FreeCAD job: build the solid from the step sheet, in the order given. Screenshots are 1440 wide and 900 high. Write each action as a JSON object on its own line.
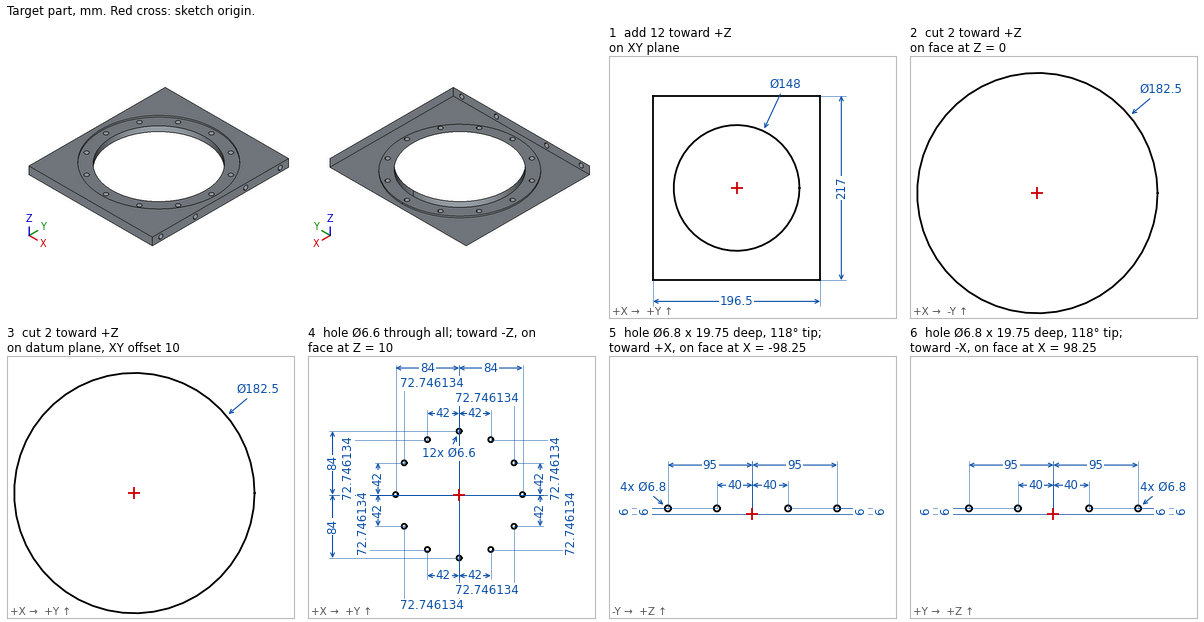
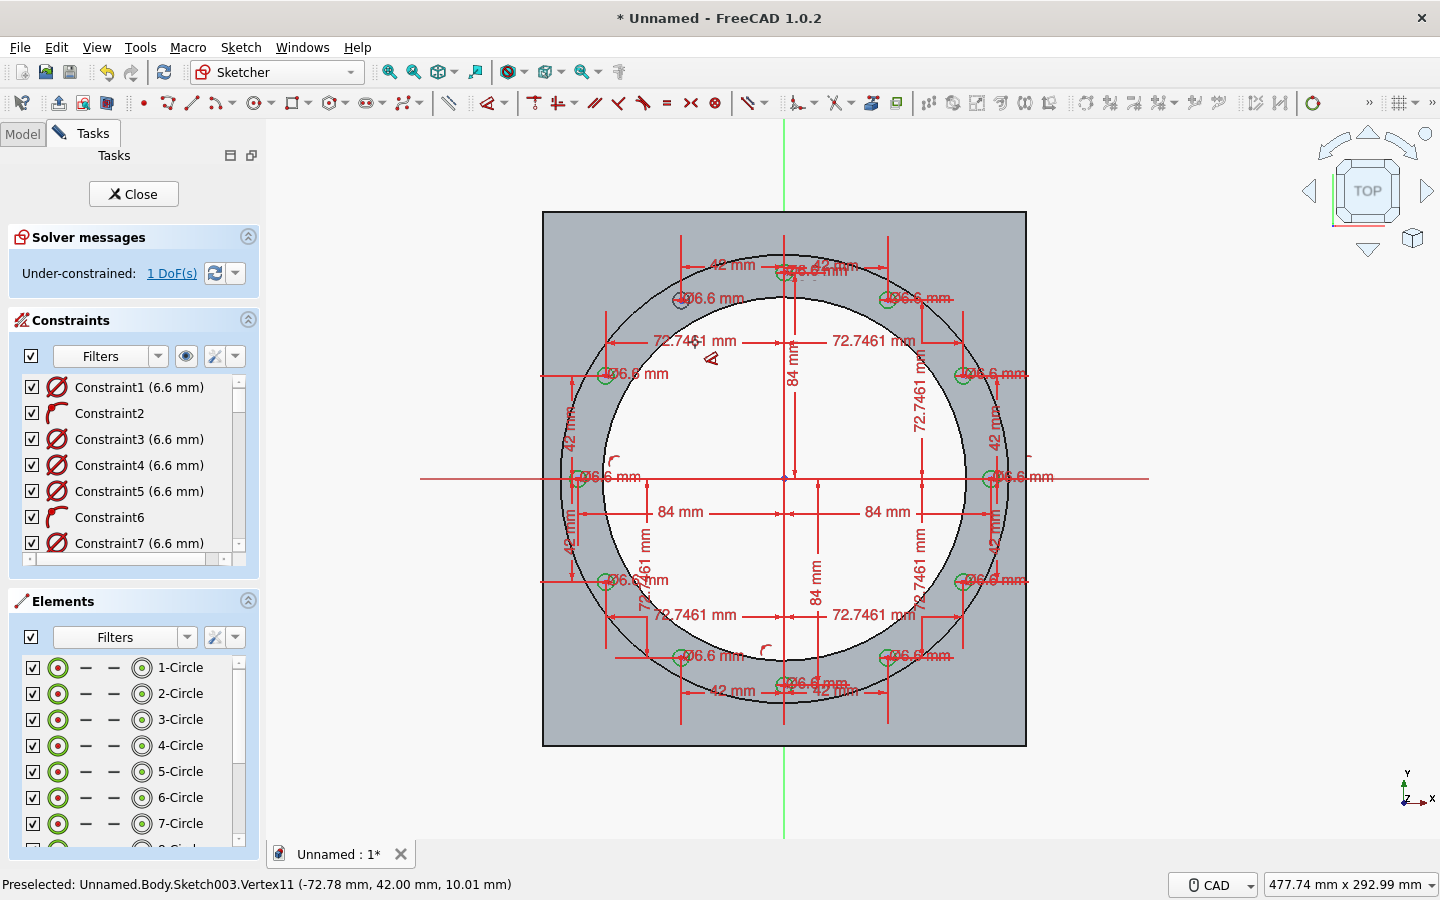
{"action": "left_click", "coordinate": [681, 300]}
{"action": "left_click", "coordinate": [647, 390]}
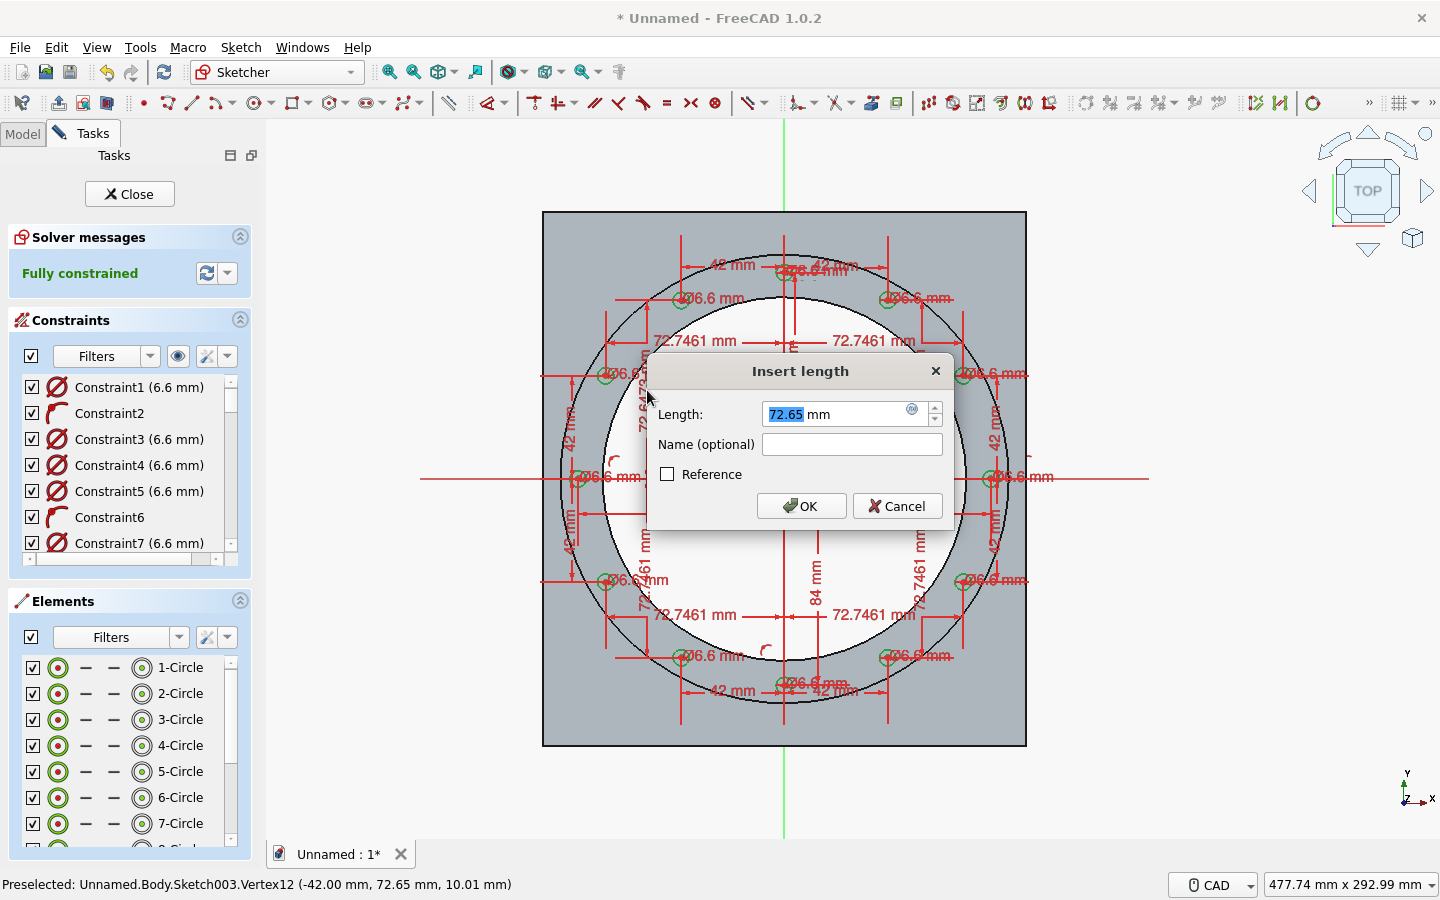
{"action": "type", "text": "72.746134"}
{"action": "key", "text": "Return"}
{"action": "key", "text": "Escape"}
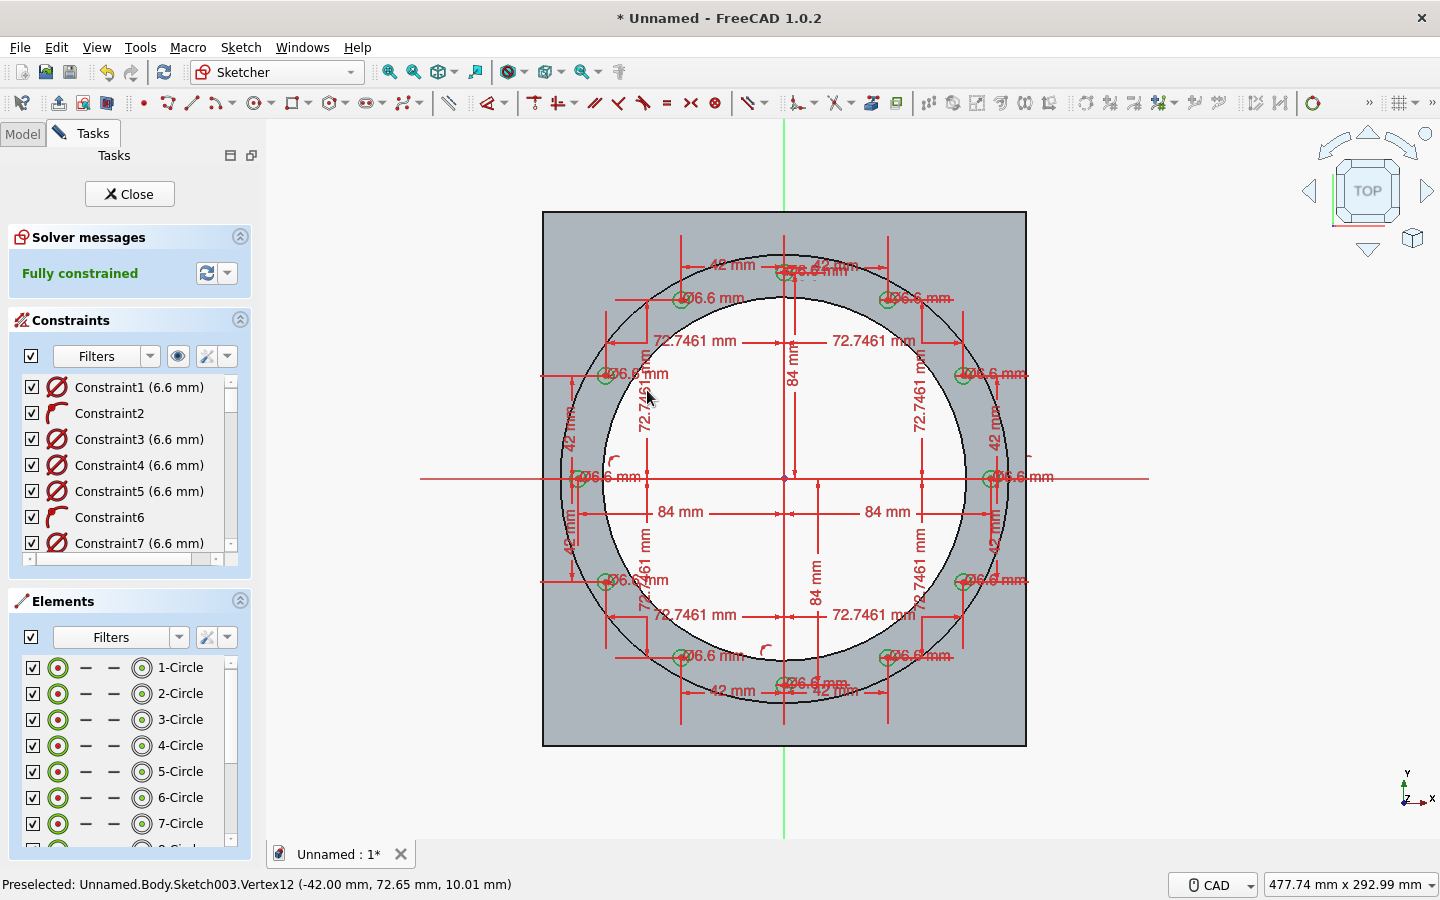
{"action": "left_click", "coordinate": [130, 194]}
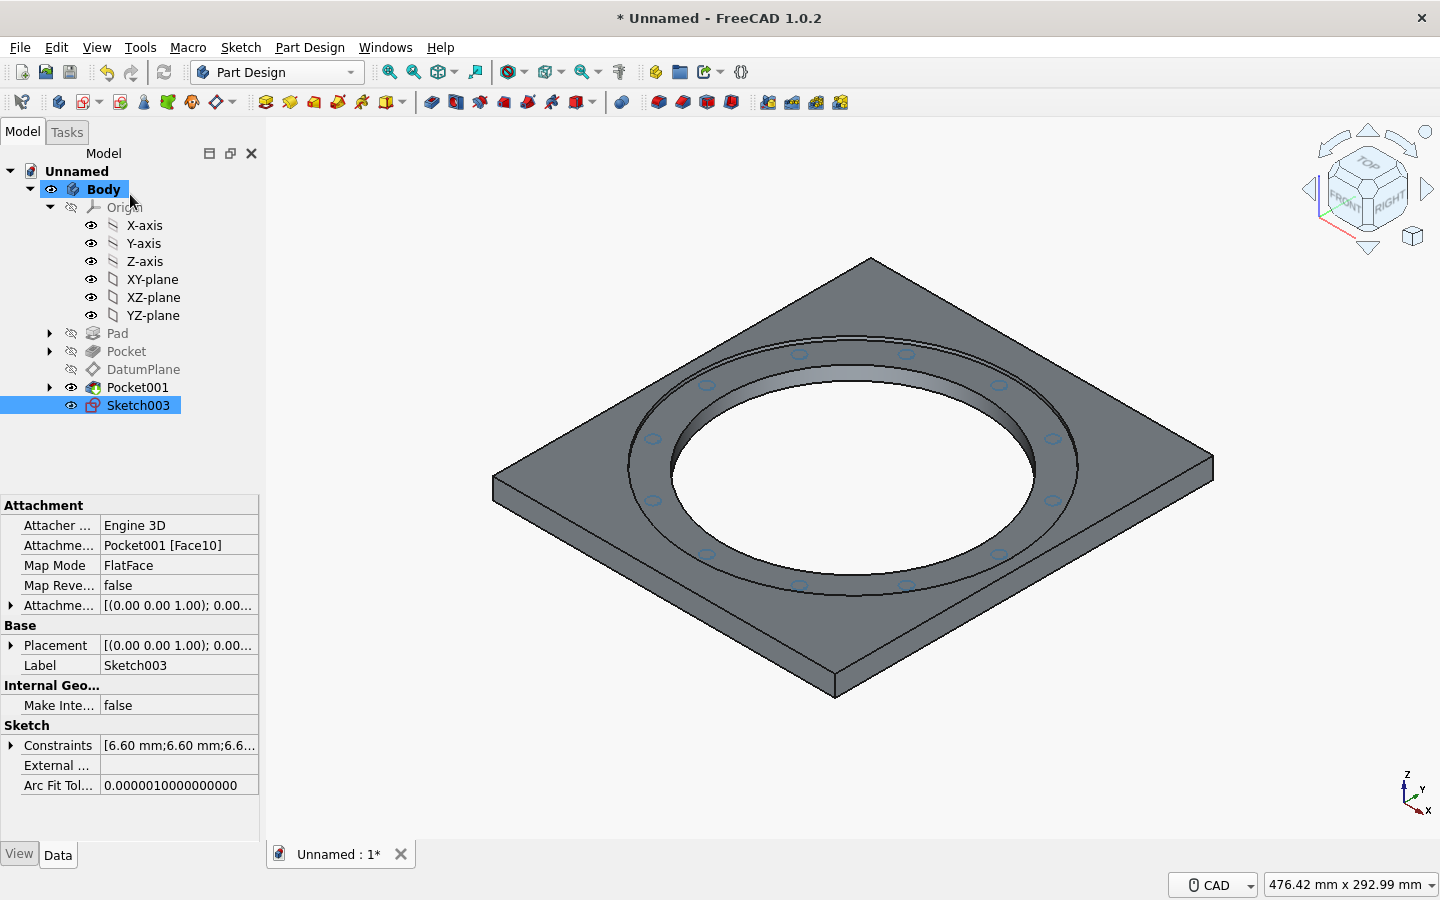
{"action": "left_click", "coordinate": [456, 102]}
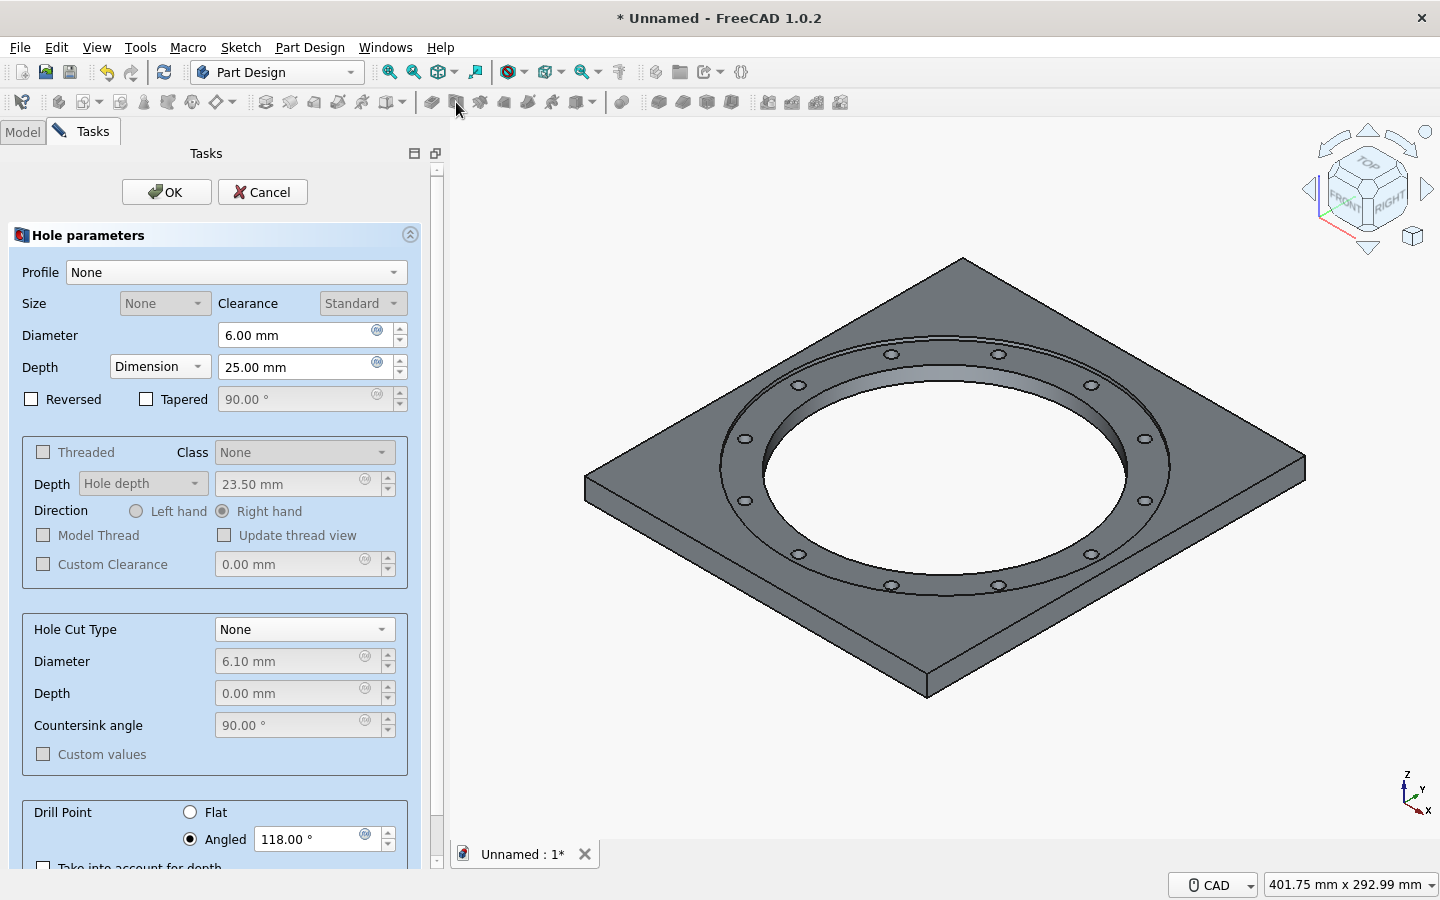
{"action": "triple_click", "coordinate": [305, 335]}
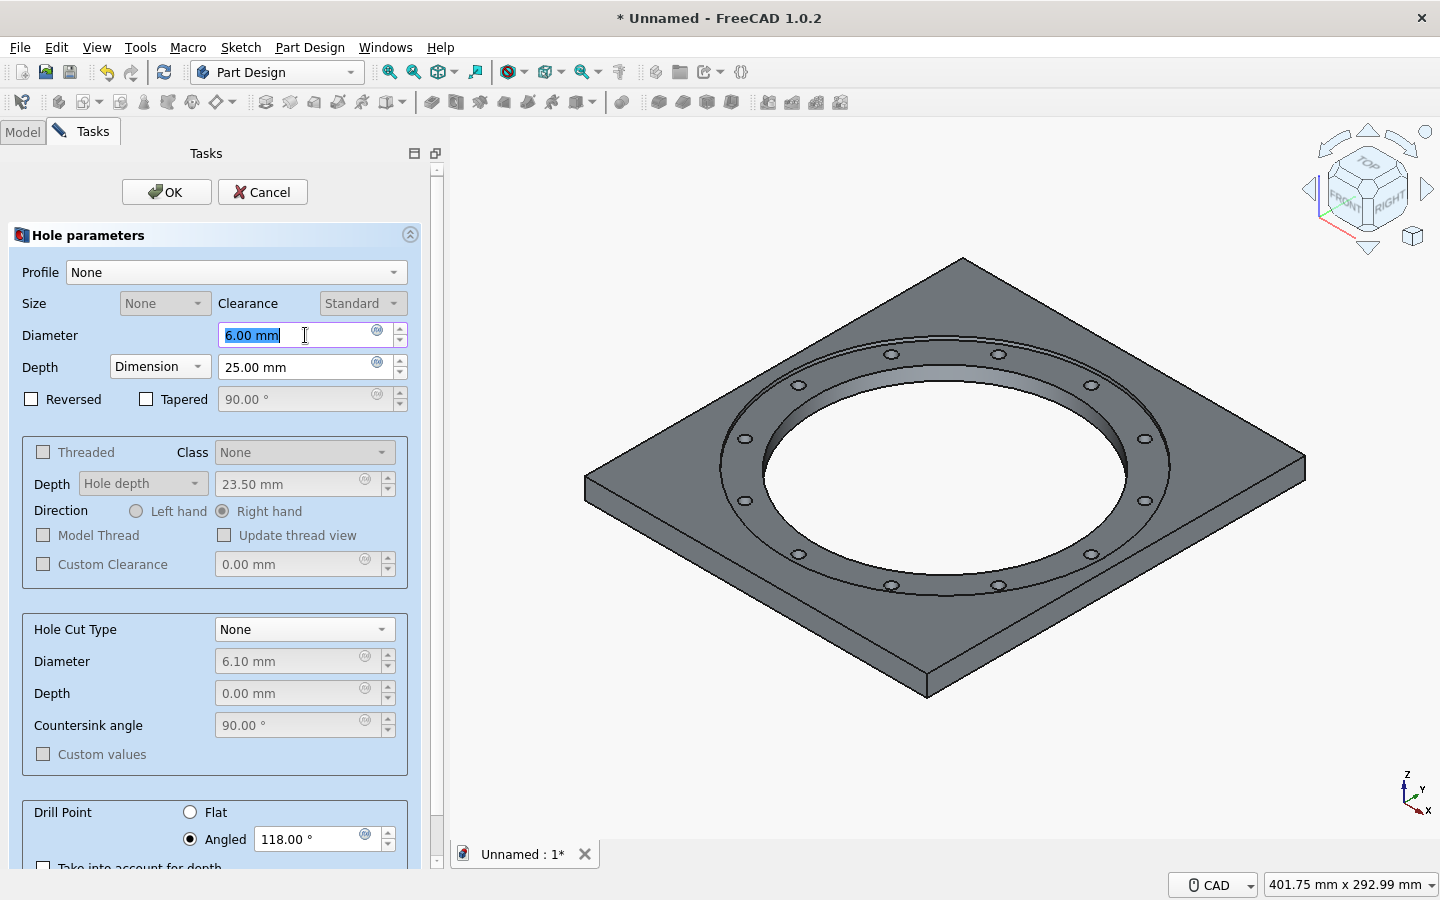
{"action": "type", "text": "6.6"}
{"action": "key", "text": "Tab"}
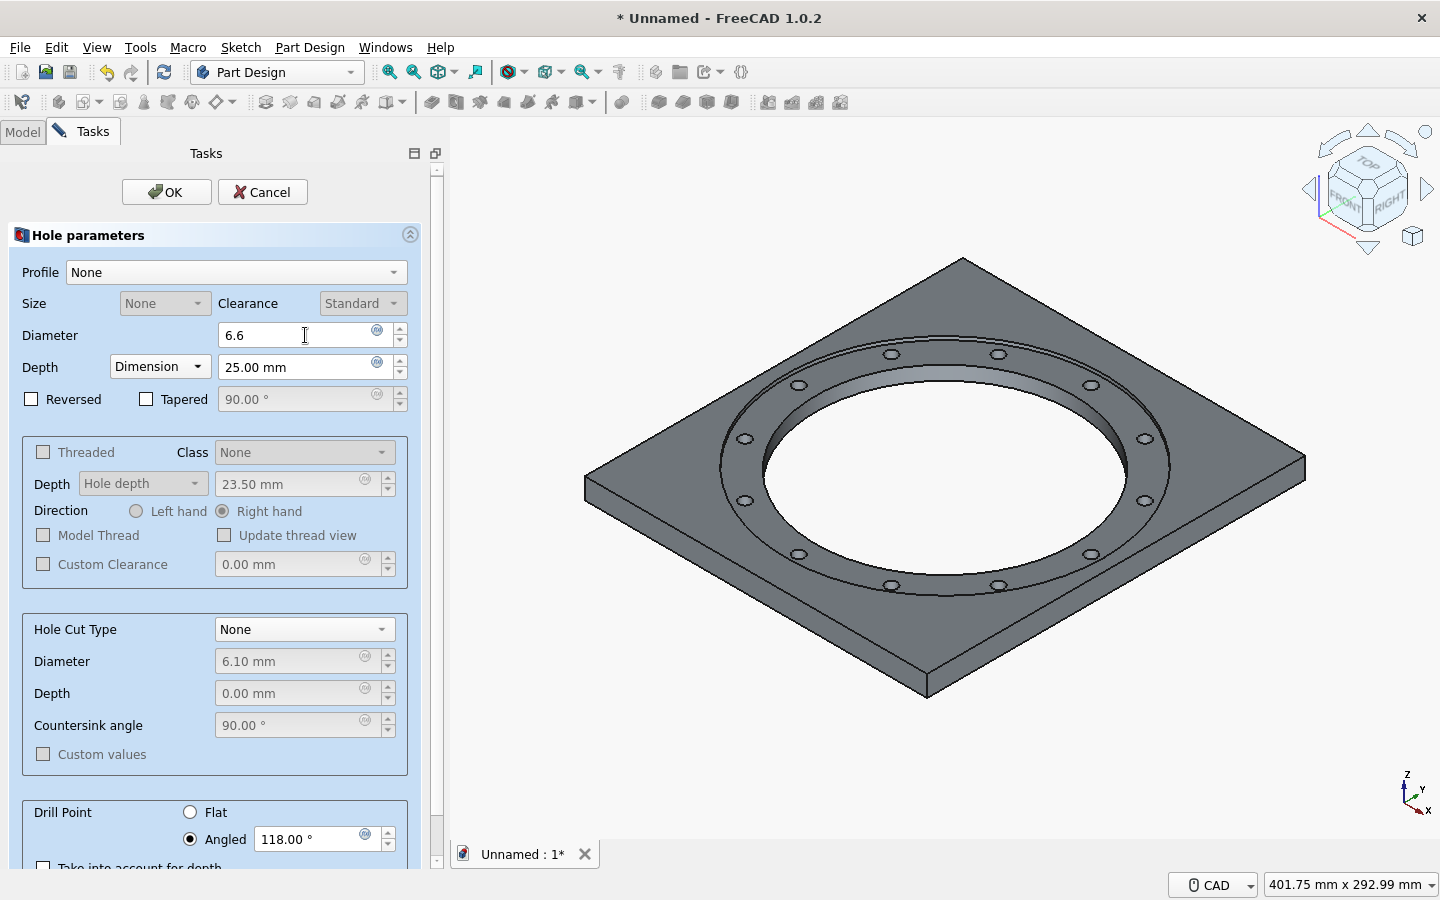
{"action": "left_click", "coordinate": [161, 366]}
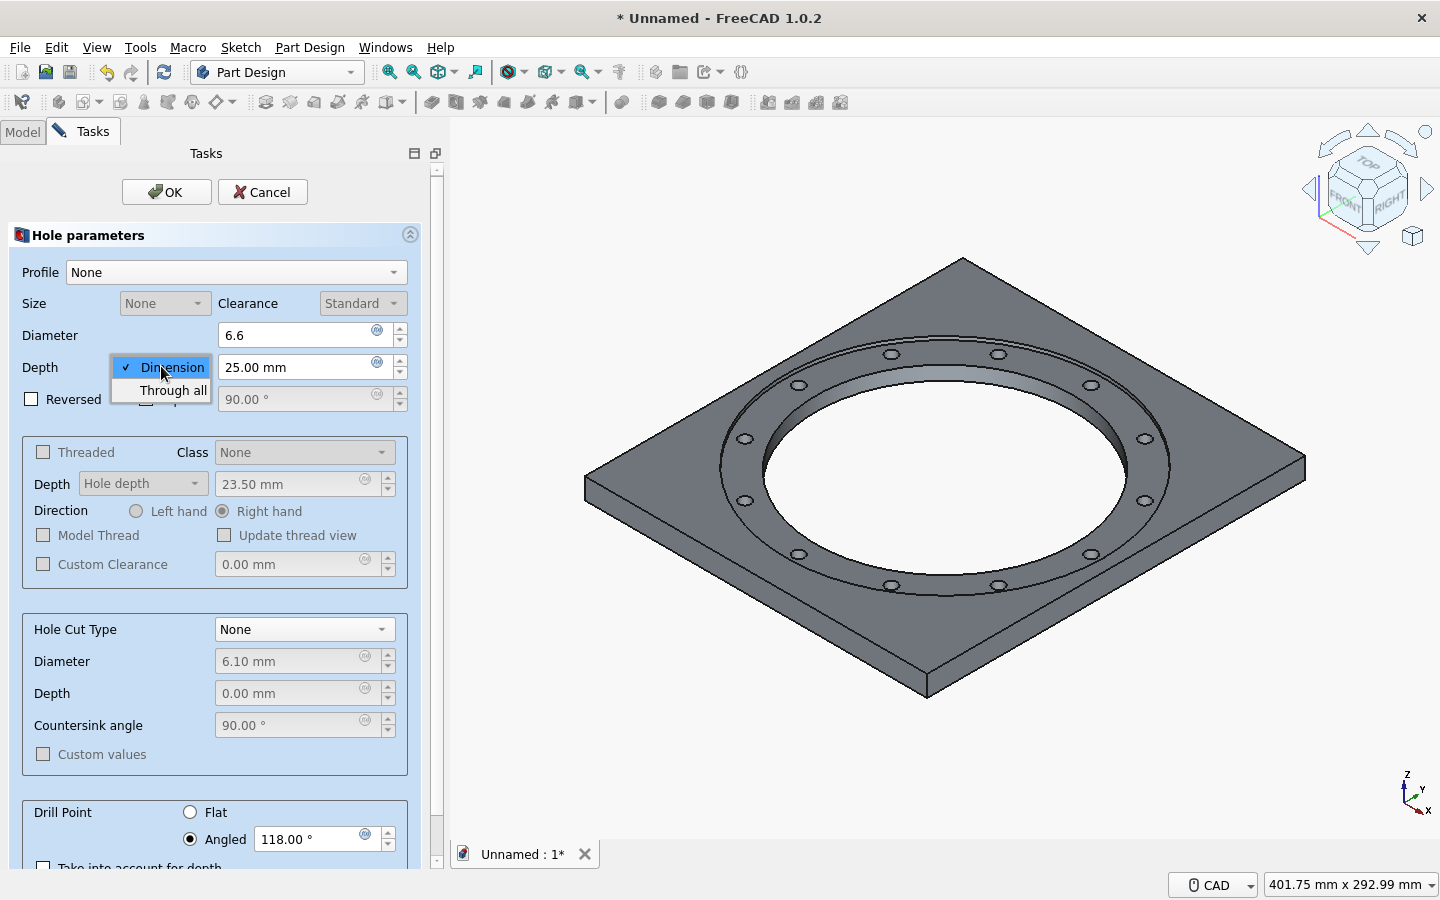
{"action": "left_click", "coordinate": [160, 390]}